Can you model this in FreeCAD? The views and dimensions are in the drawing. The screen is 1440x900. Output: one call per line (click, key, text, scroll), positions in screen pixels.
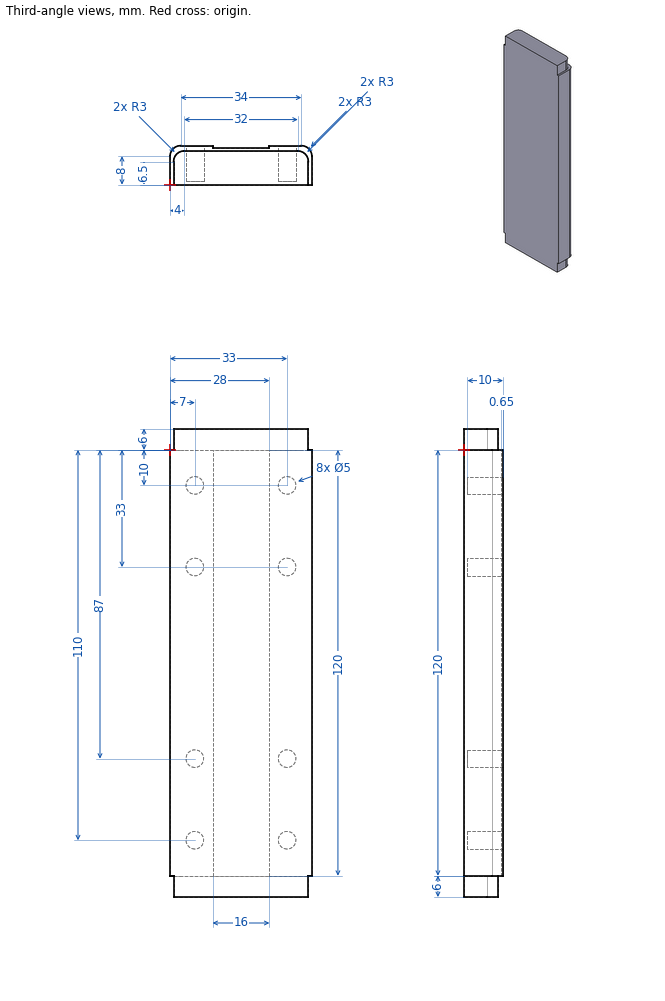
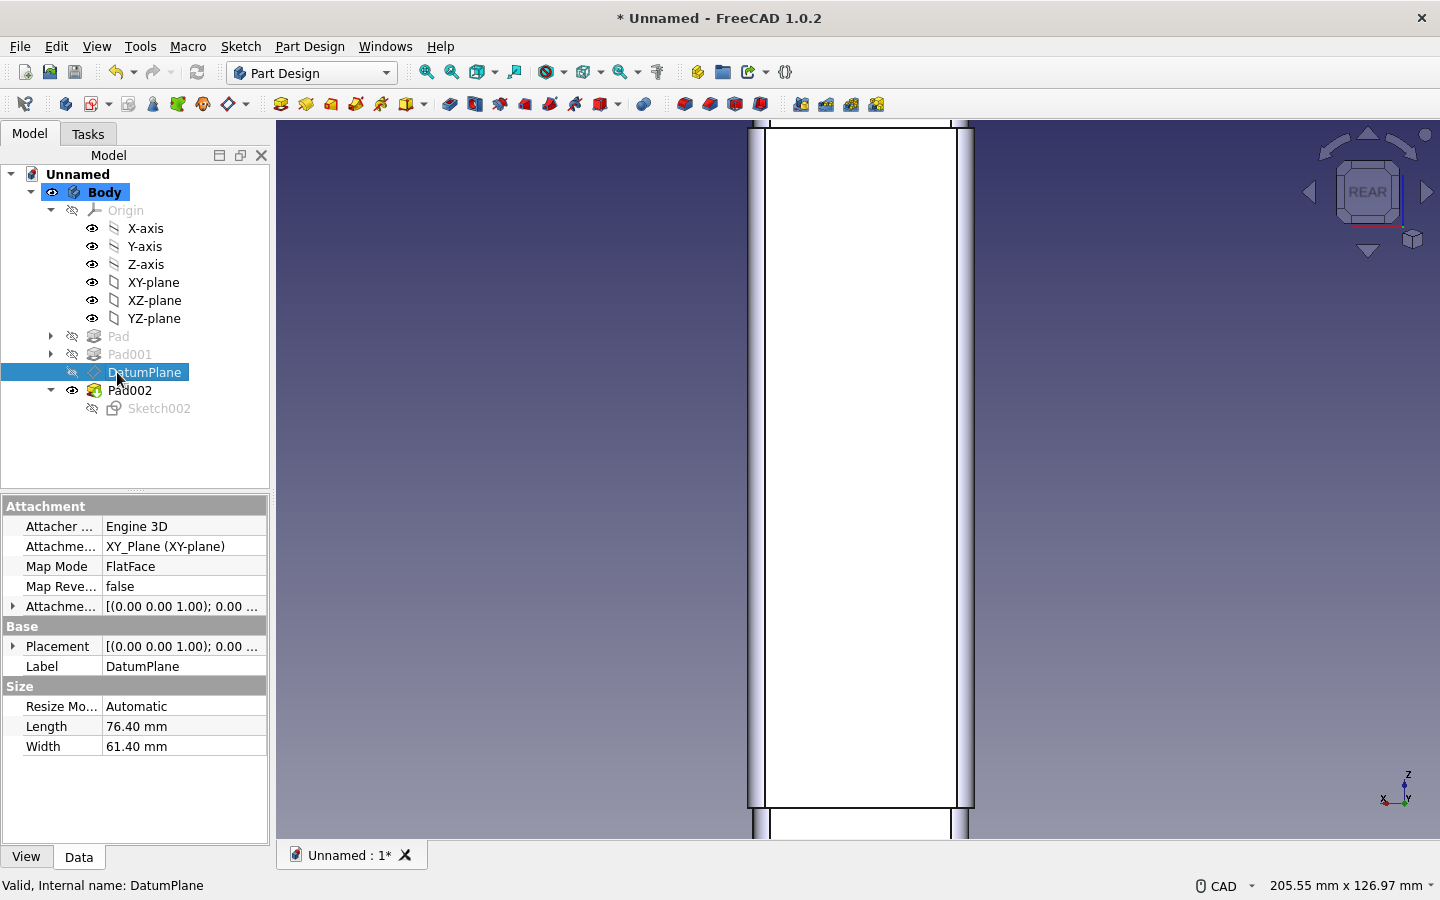
click(427, 72)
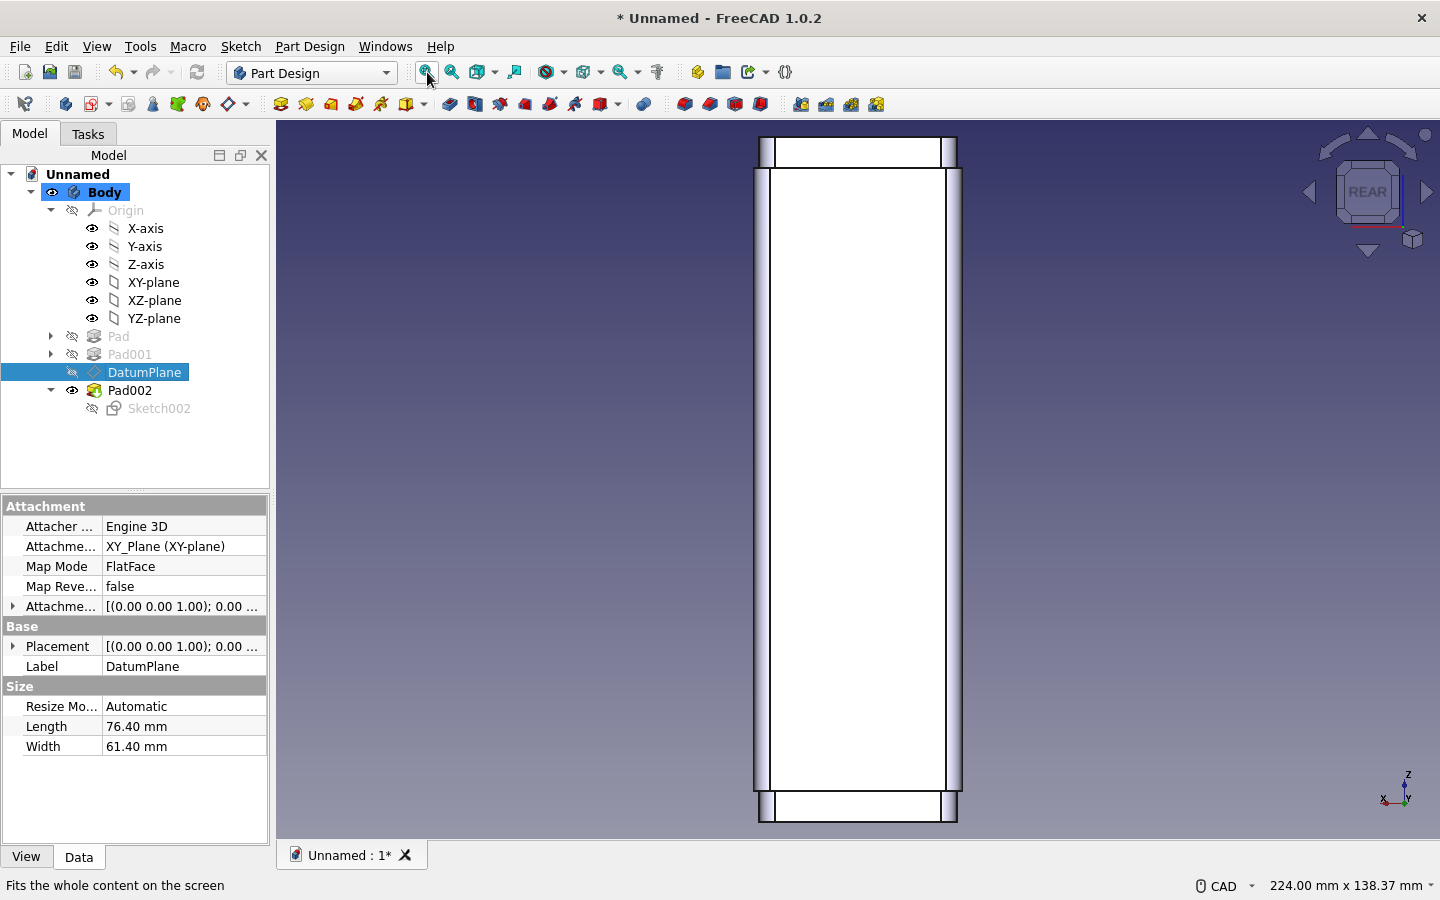
click(858, 300)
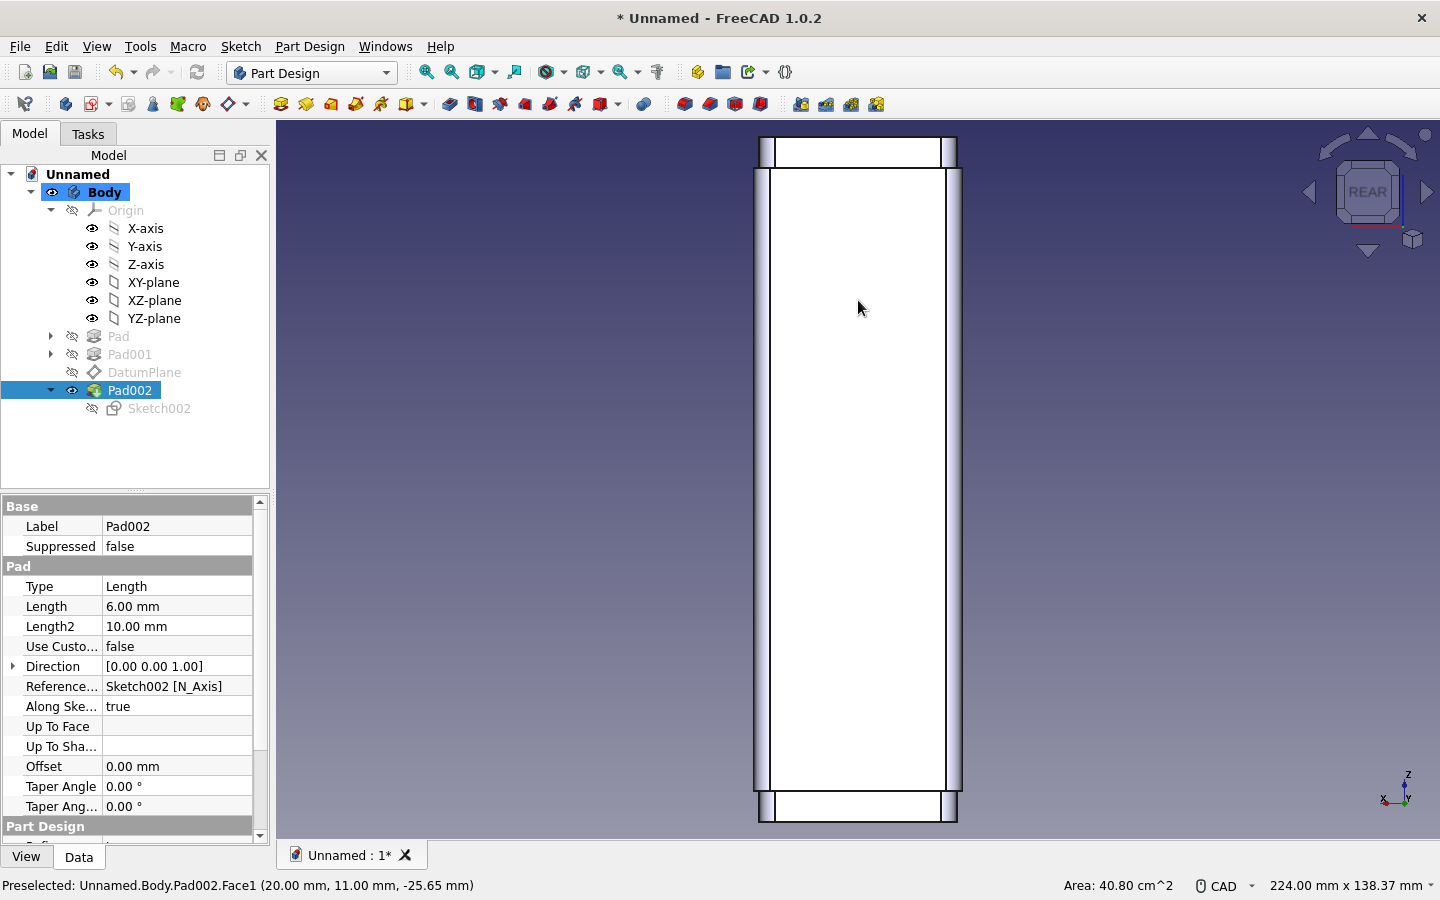
click(90, 104)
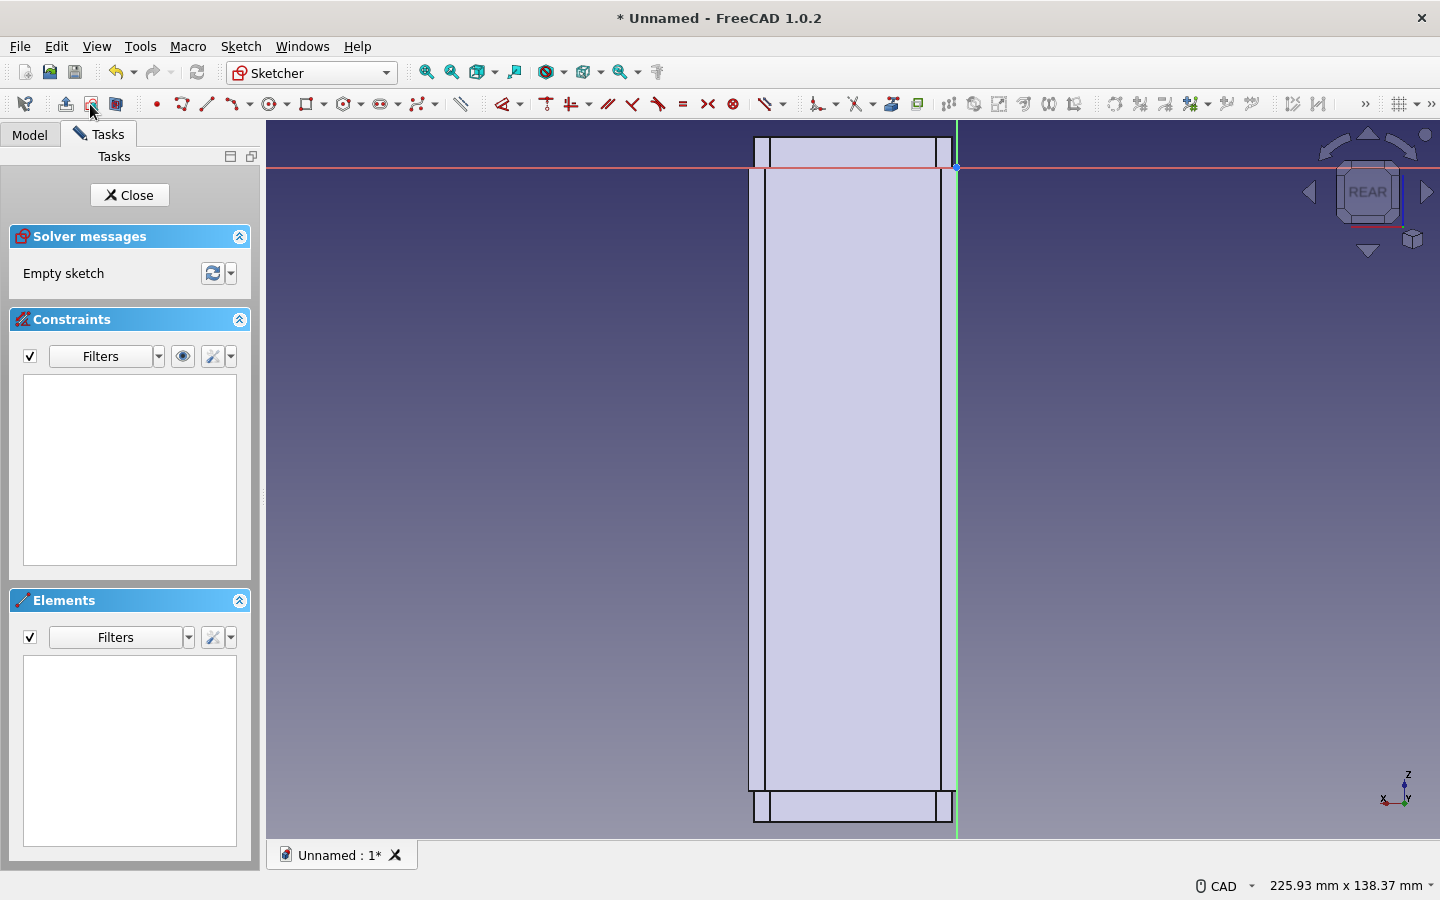
scroll(422, 568, down, 1)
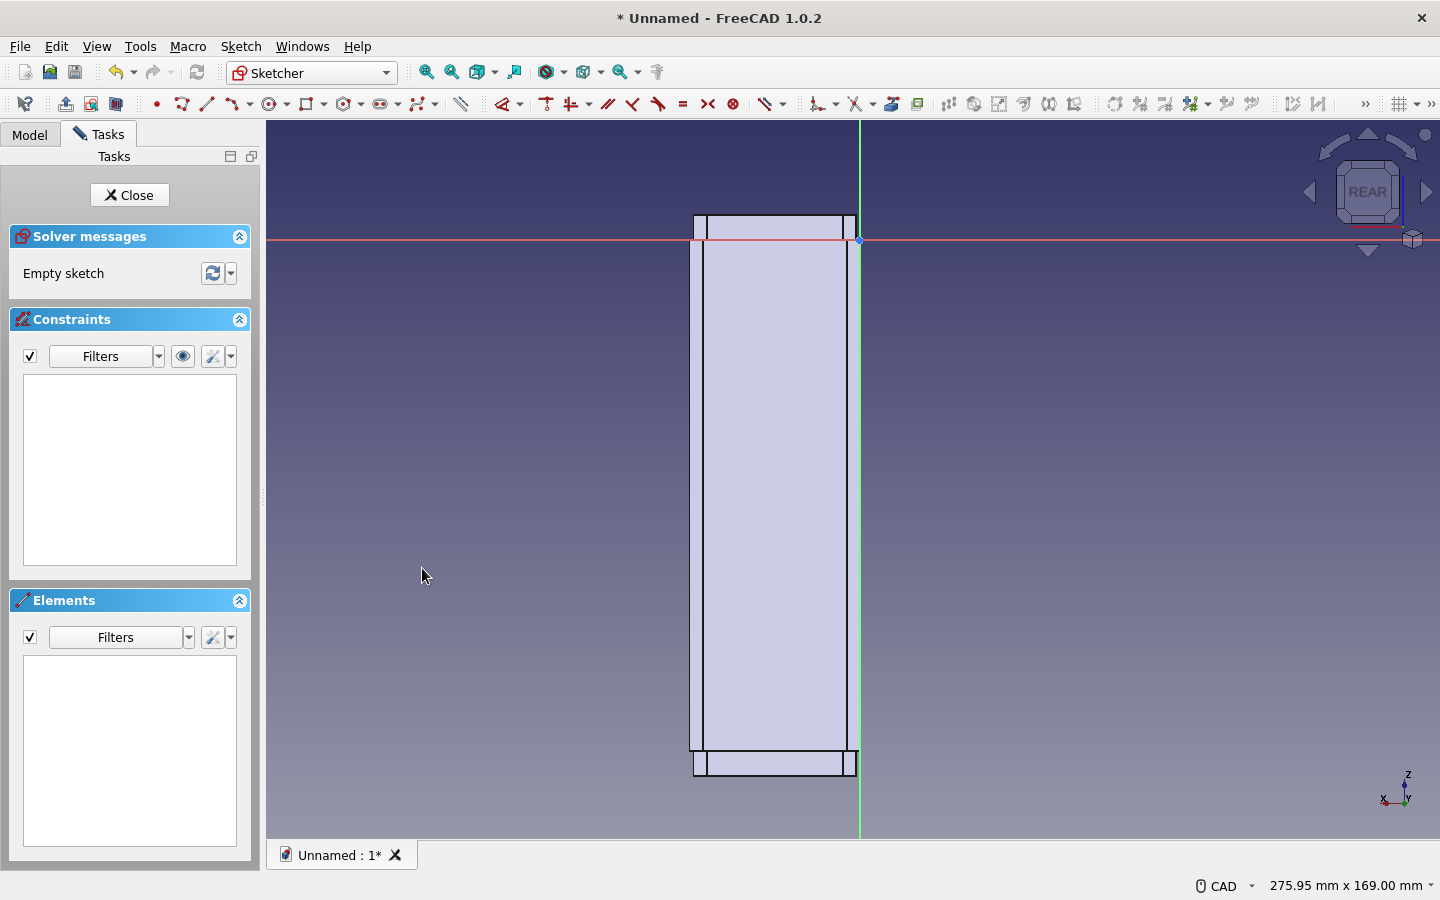
key(g)
key(c)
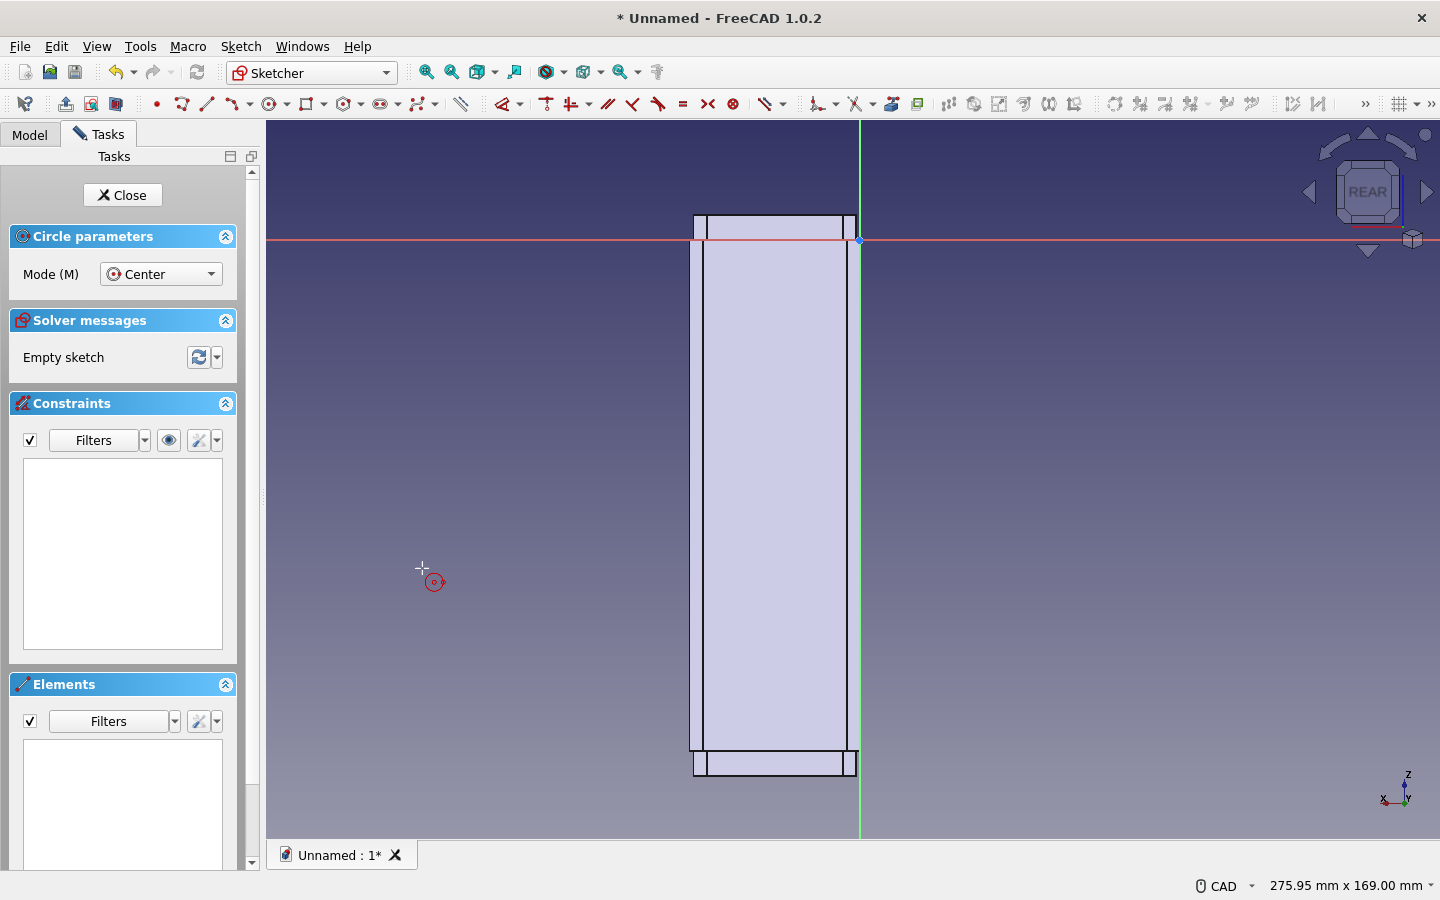
scroll(720, 283, up, 4)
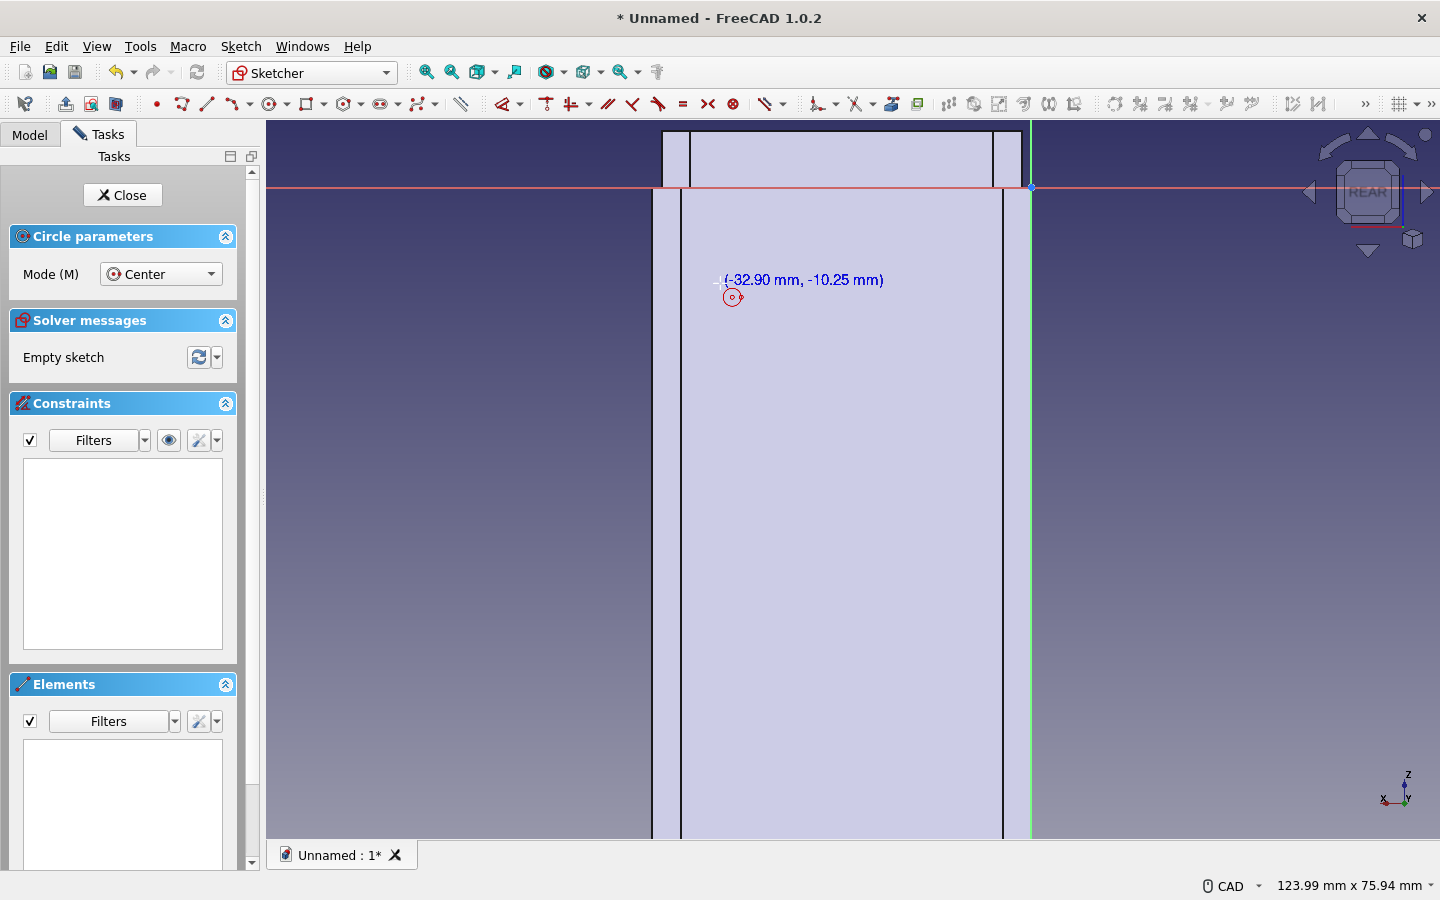
click(719, 283)
click(735, 266)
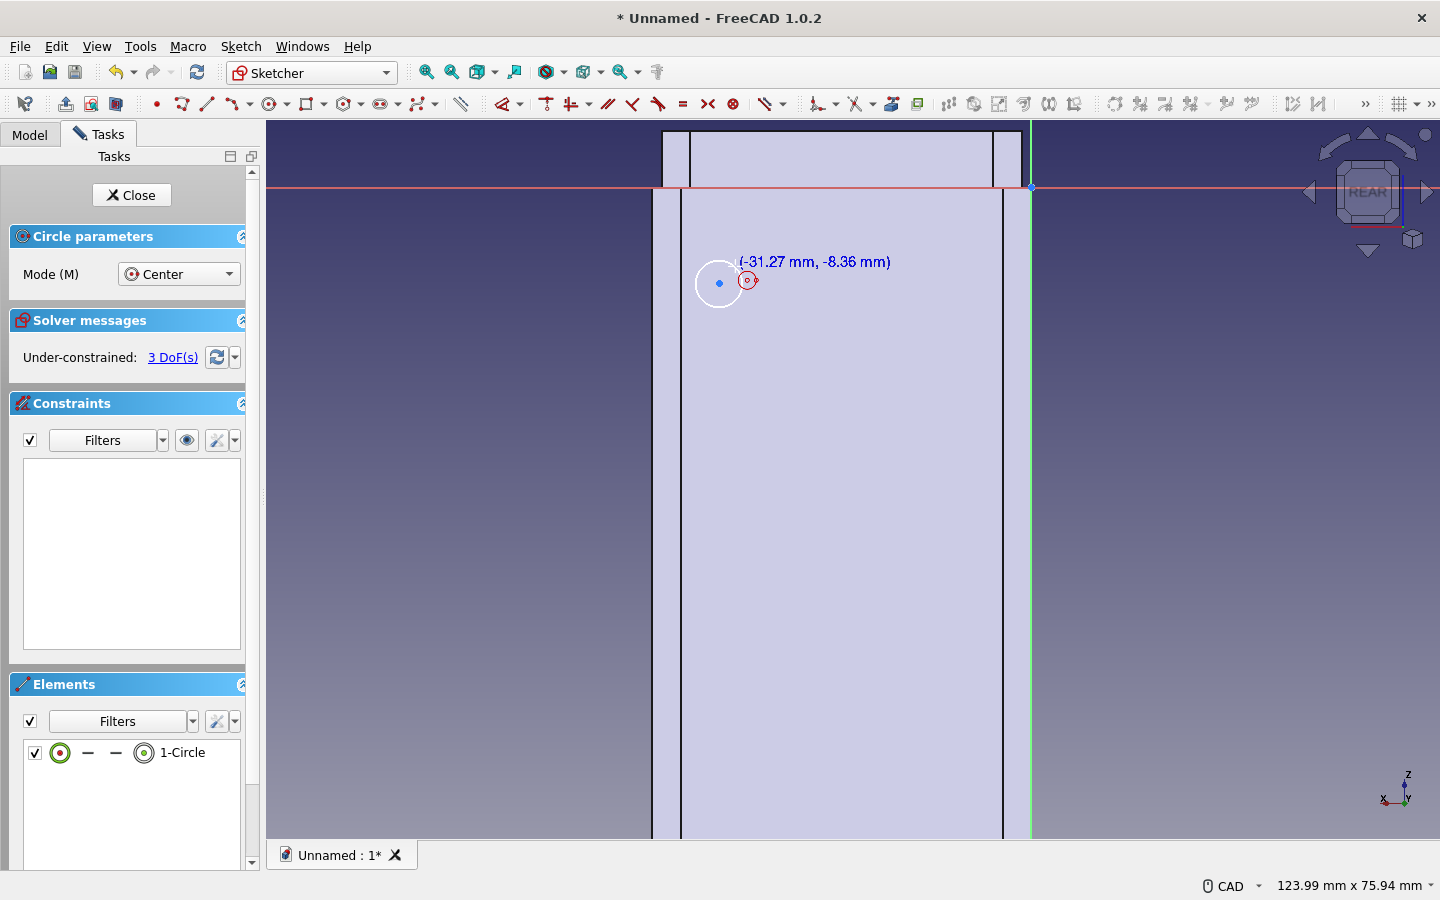
click(965, 283)
click(982, 266)